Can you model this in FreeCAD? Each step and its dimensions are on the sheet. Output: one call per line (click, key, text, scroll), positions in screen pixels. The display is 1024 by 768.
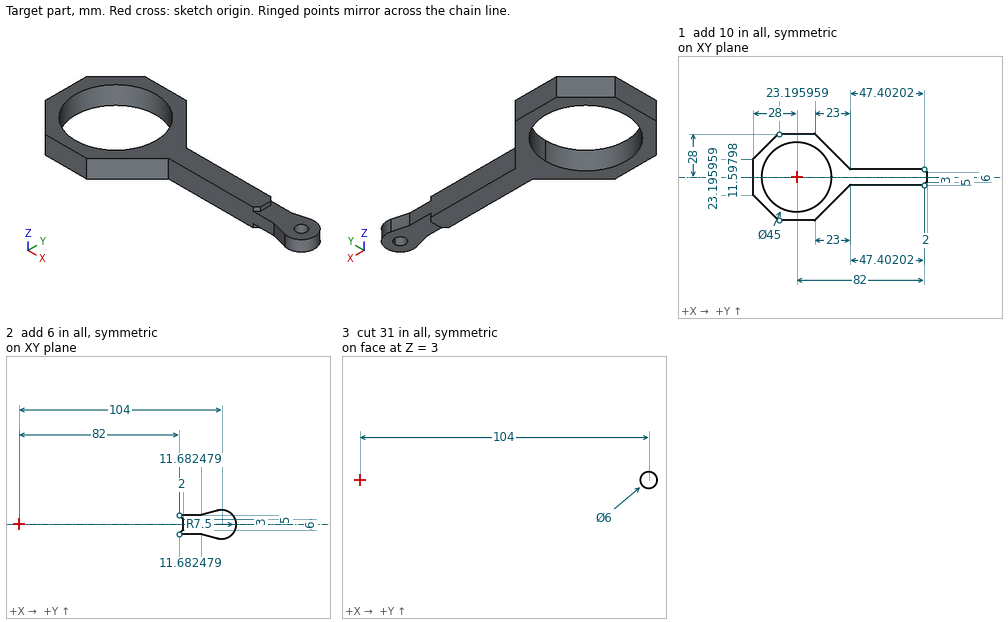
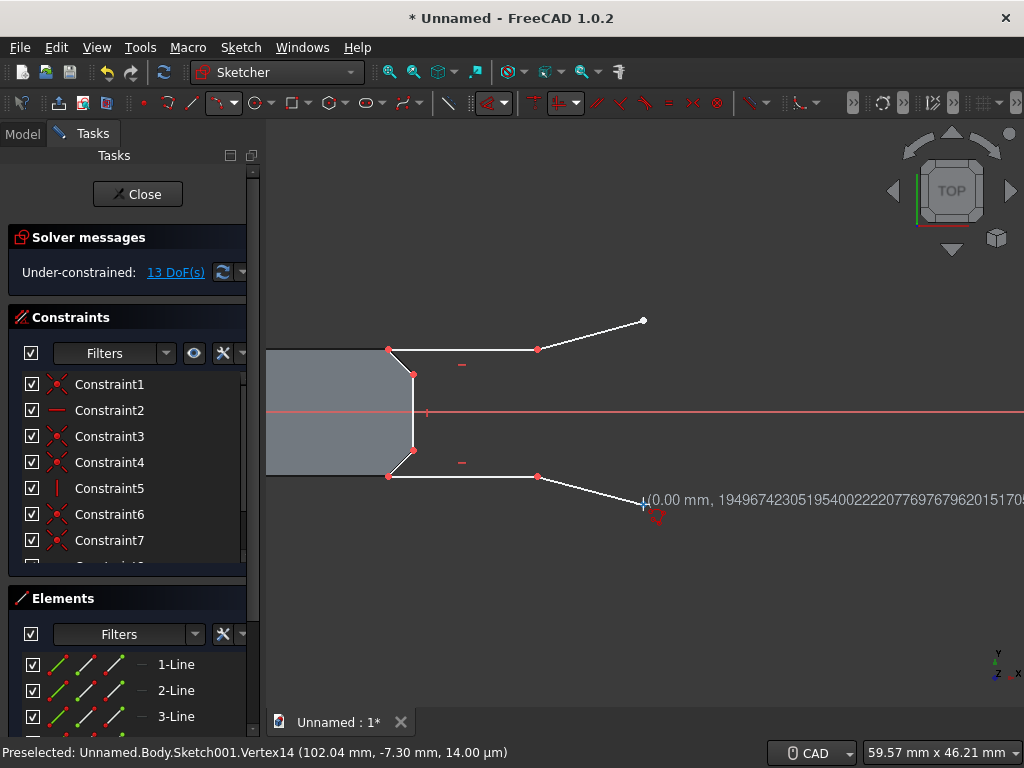
click(218, 104)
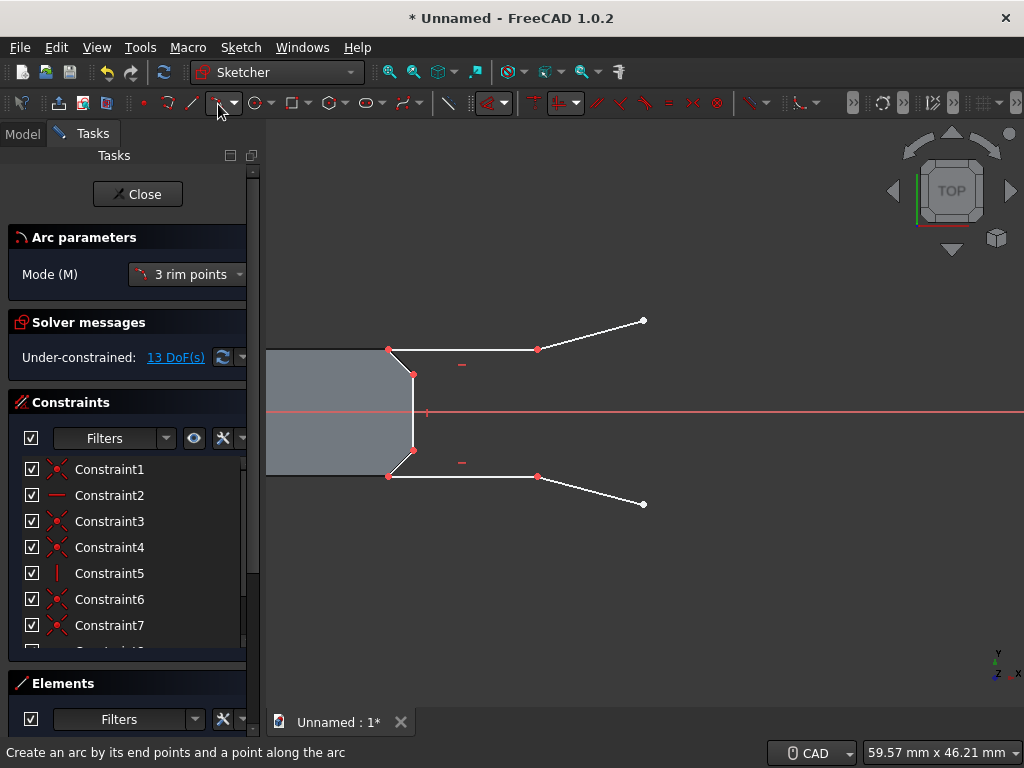
click(643, 505)
click(643, 321)
click(757, 446)
key(Escape)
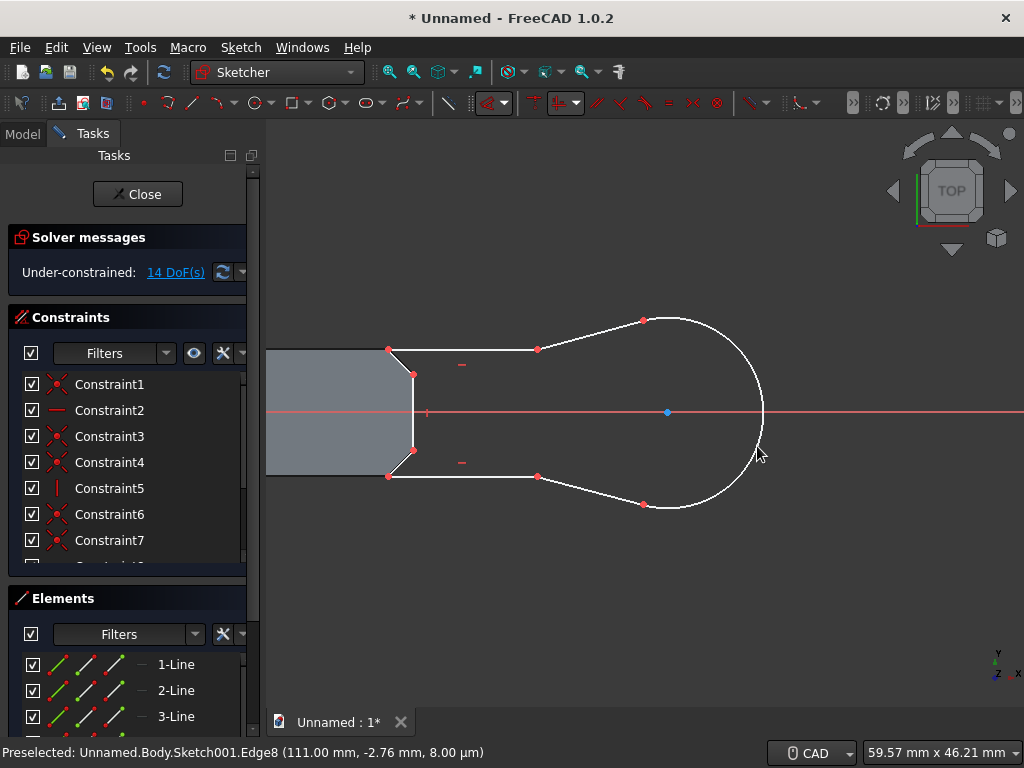
click(611, 330)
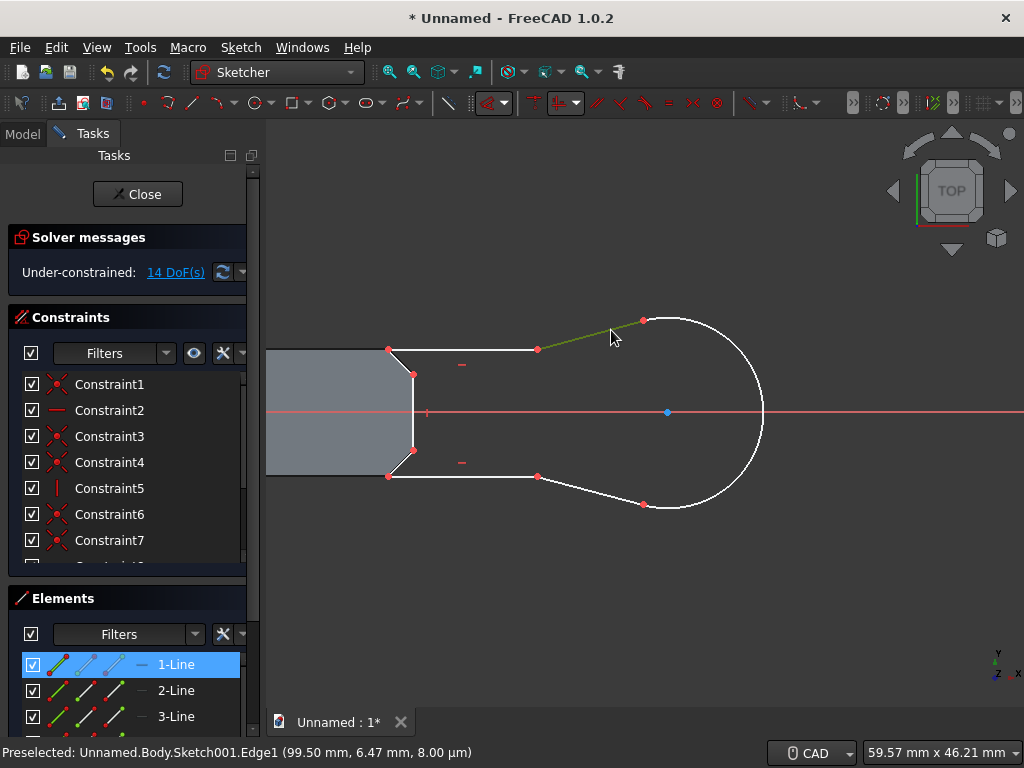
click(739, 477)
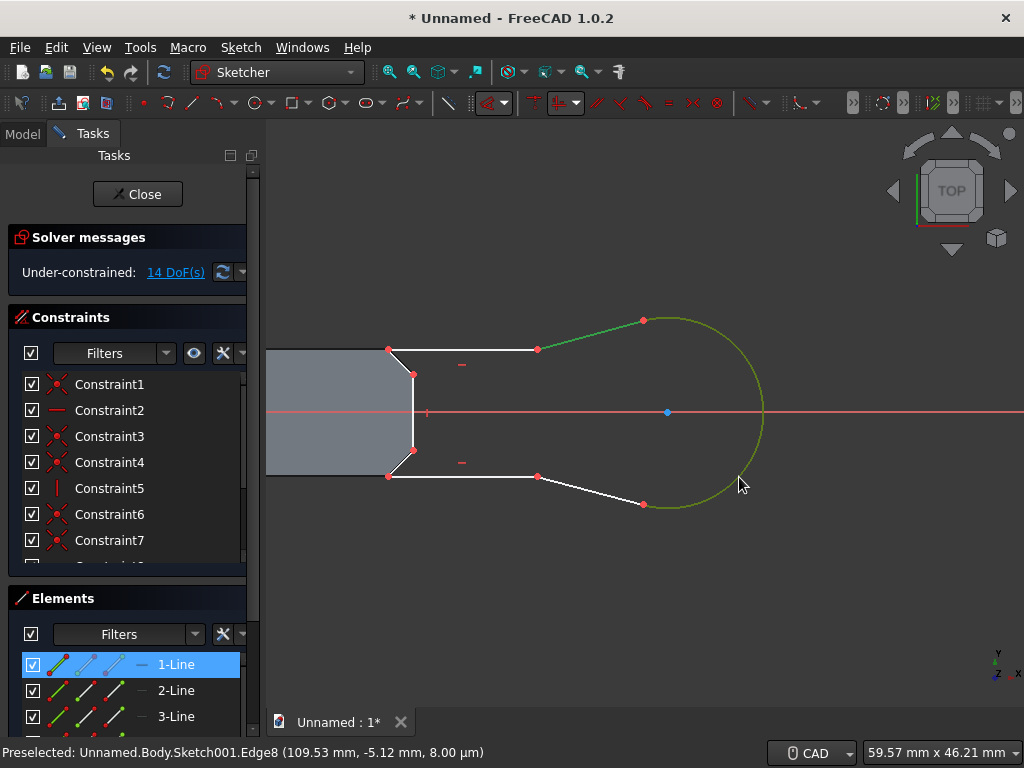
click(646, 104)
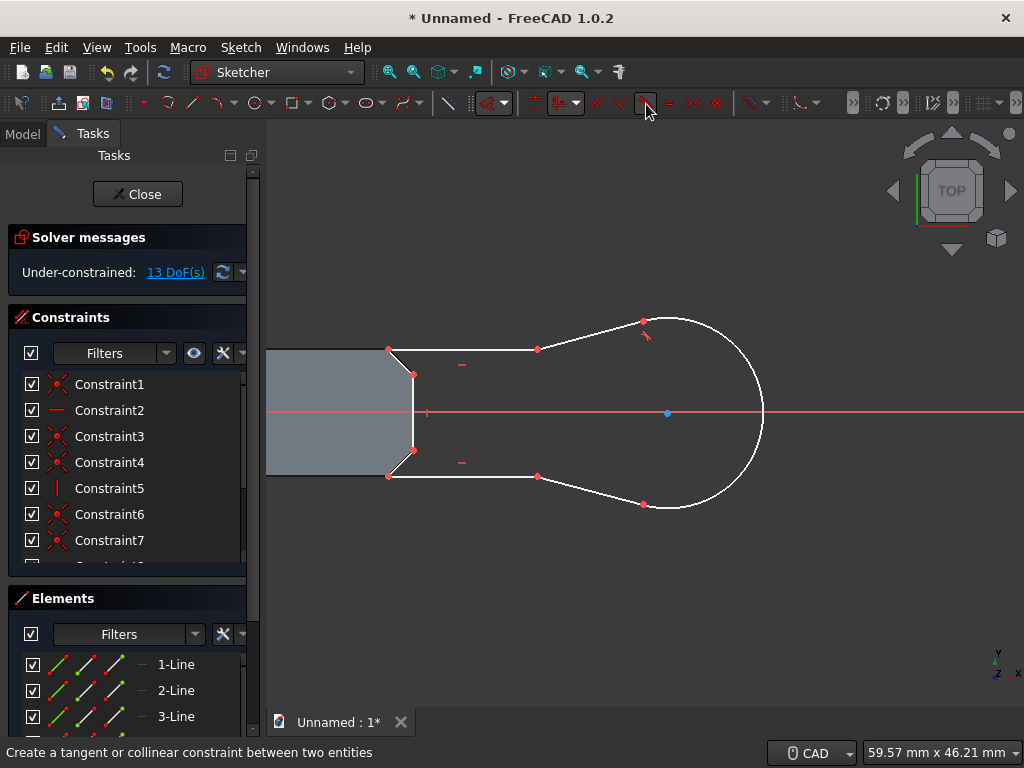
click(569, 485)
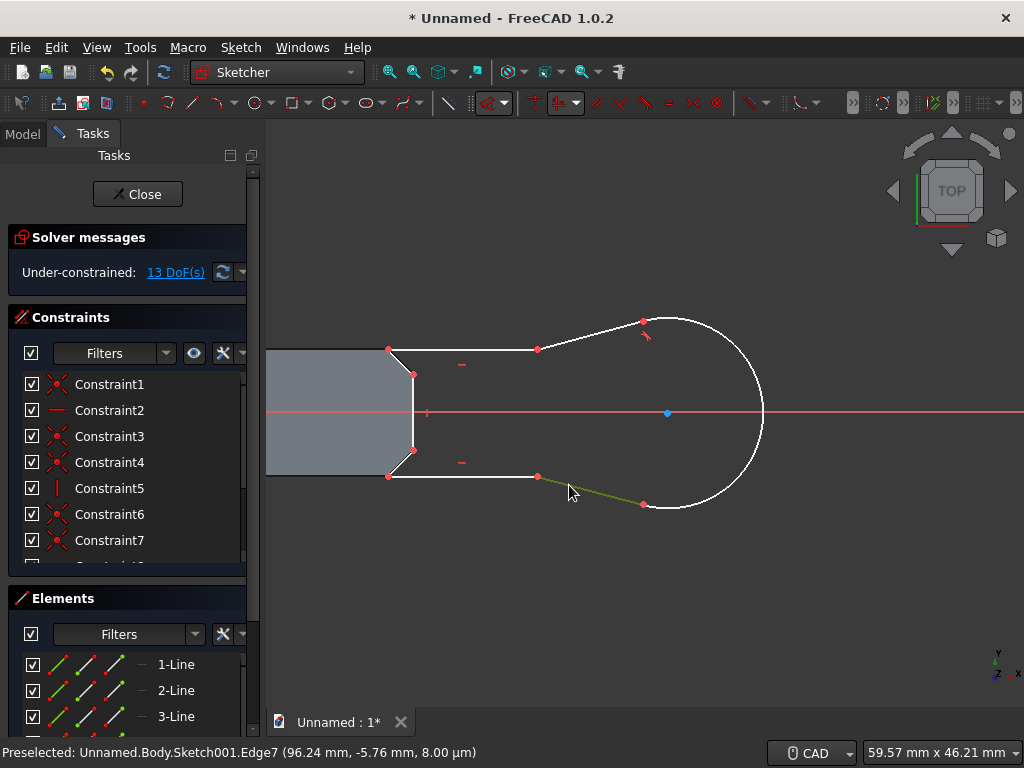
click(739, 477)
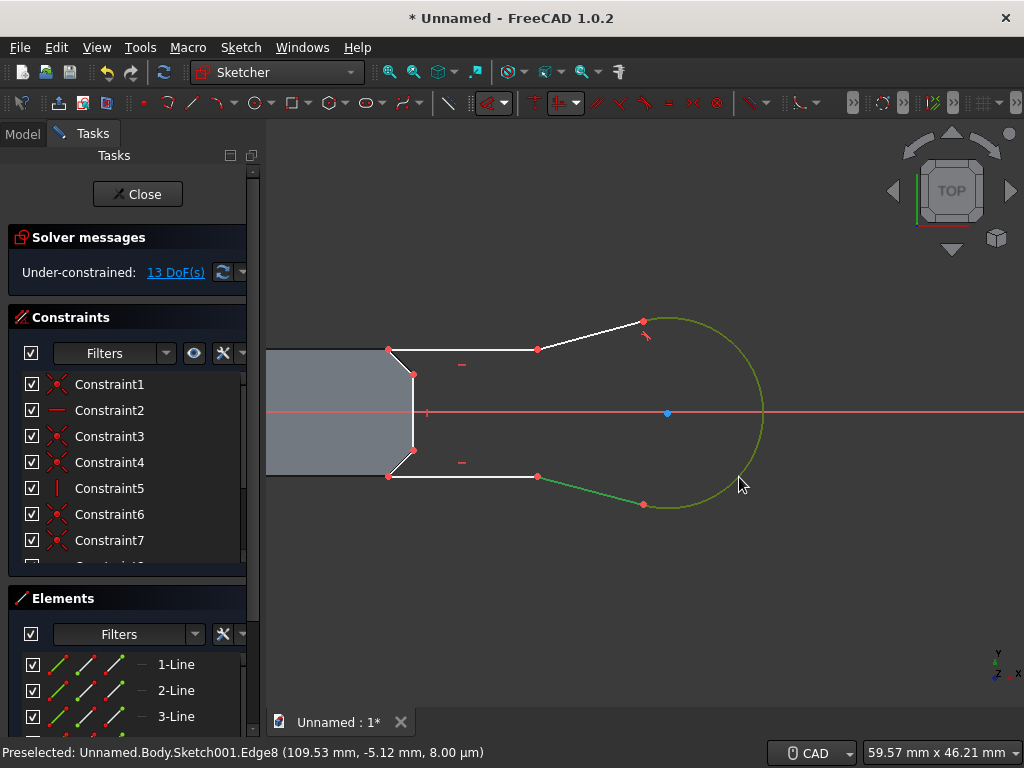
click(646, 104)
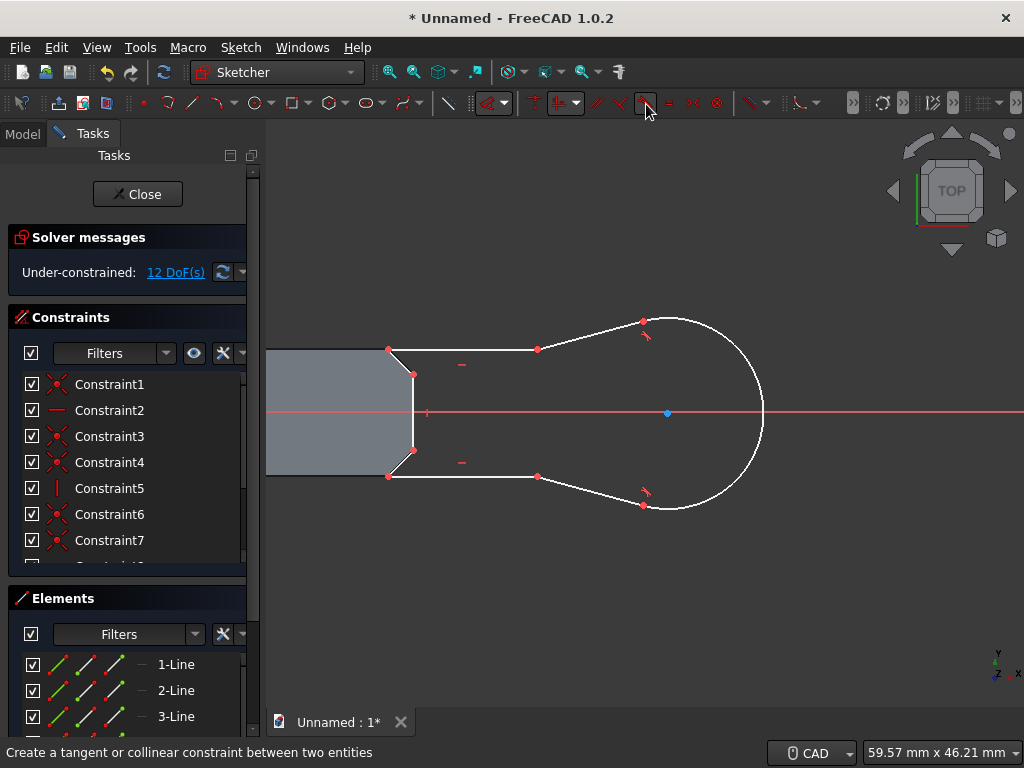
click(668, 414)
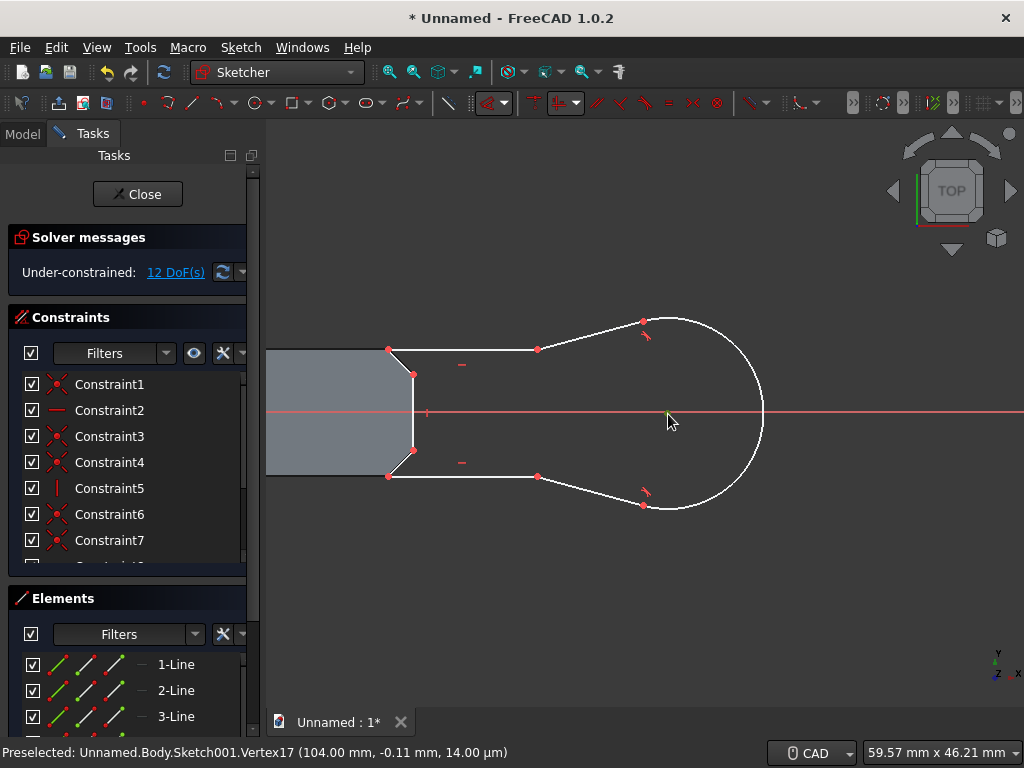
click(334, 412)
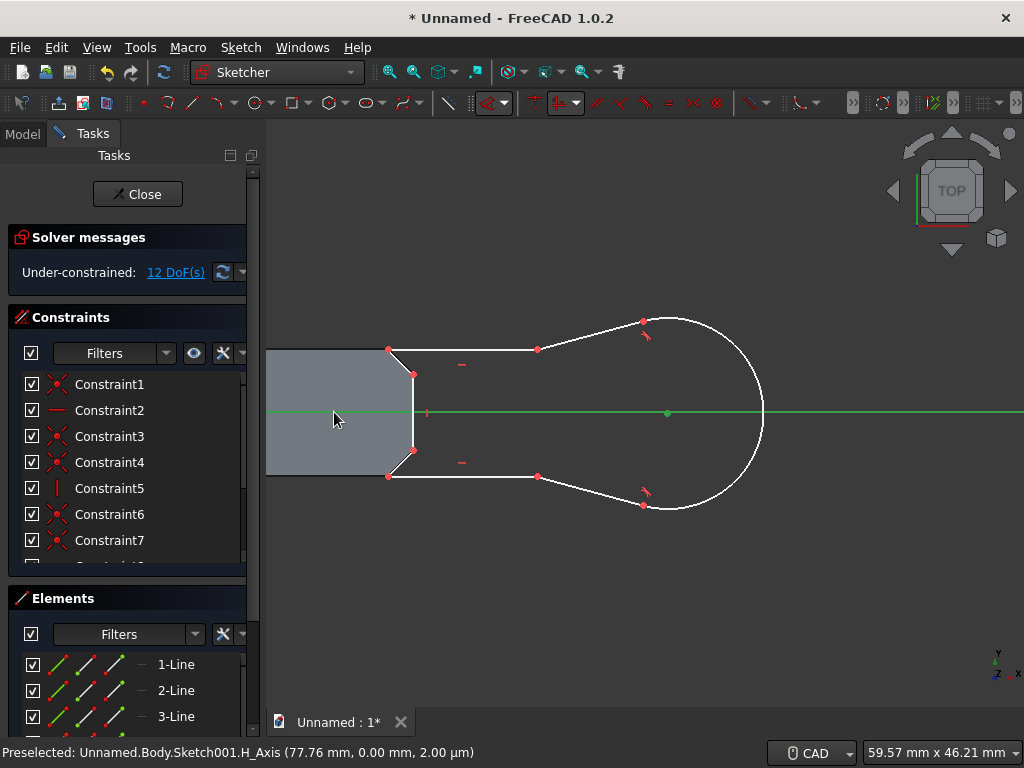
click(534, 104)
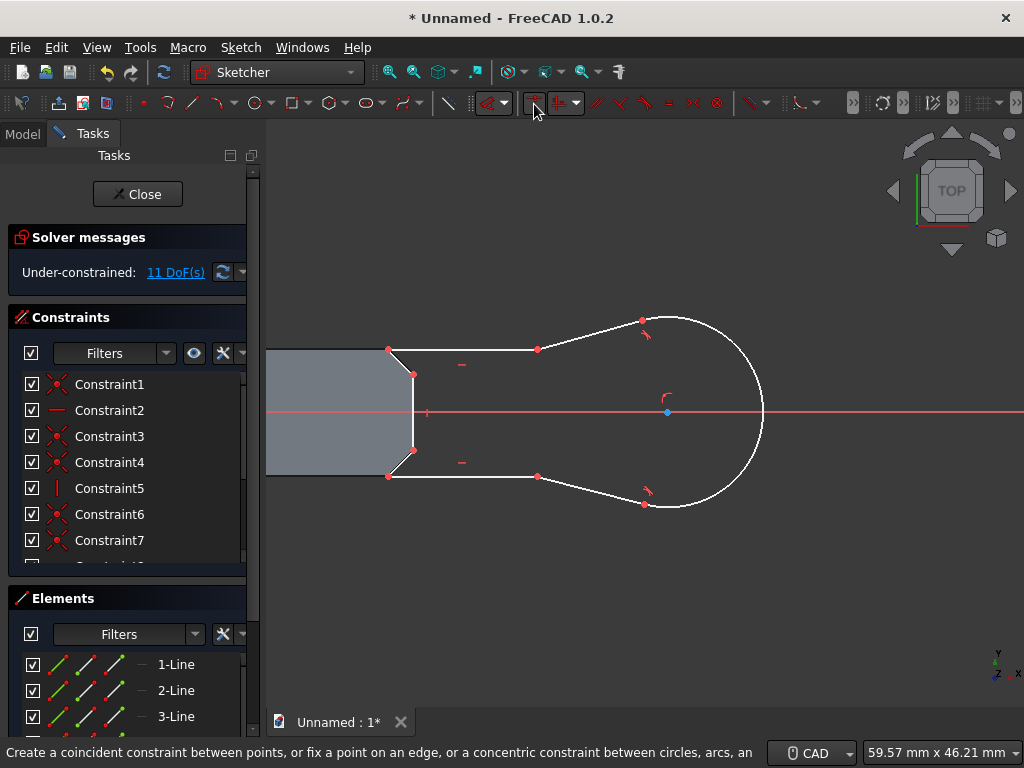
click(388, 350)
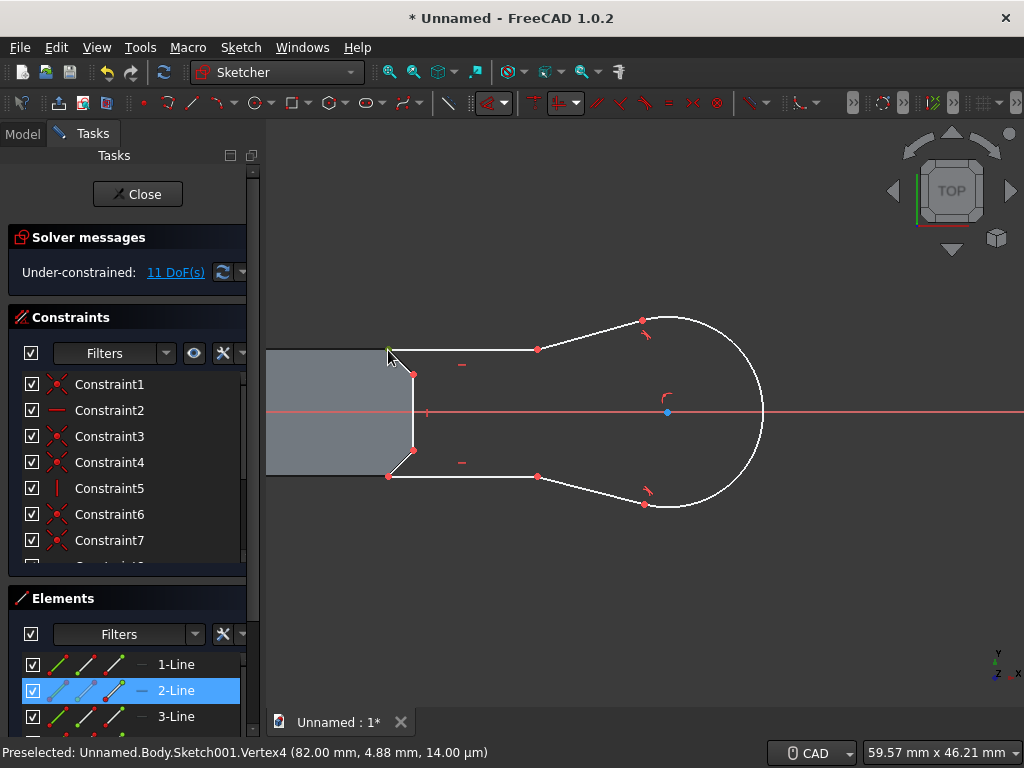
click(388, 477)